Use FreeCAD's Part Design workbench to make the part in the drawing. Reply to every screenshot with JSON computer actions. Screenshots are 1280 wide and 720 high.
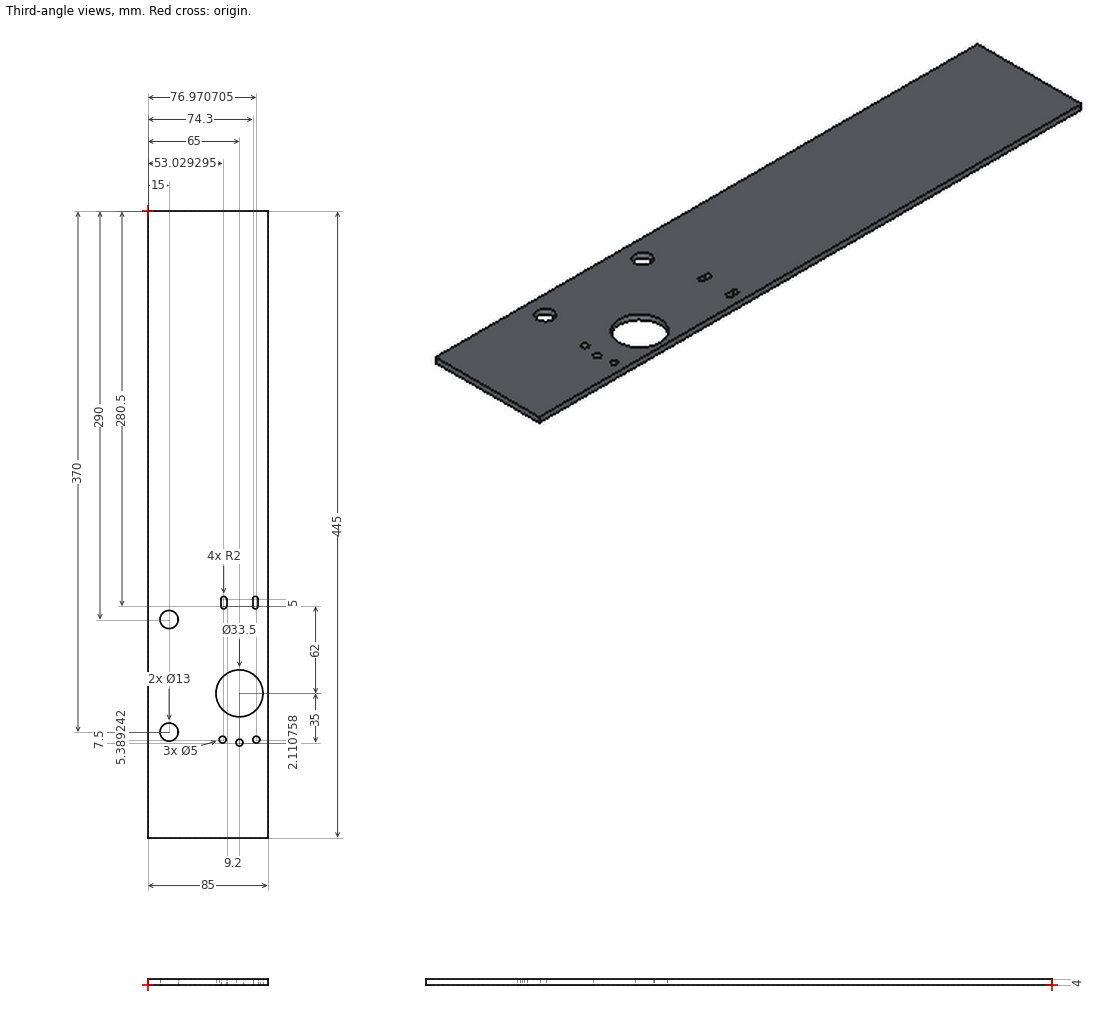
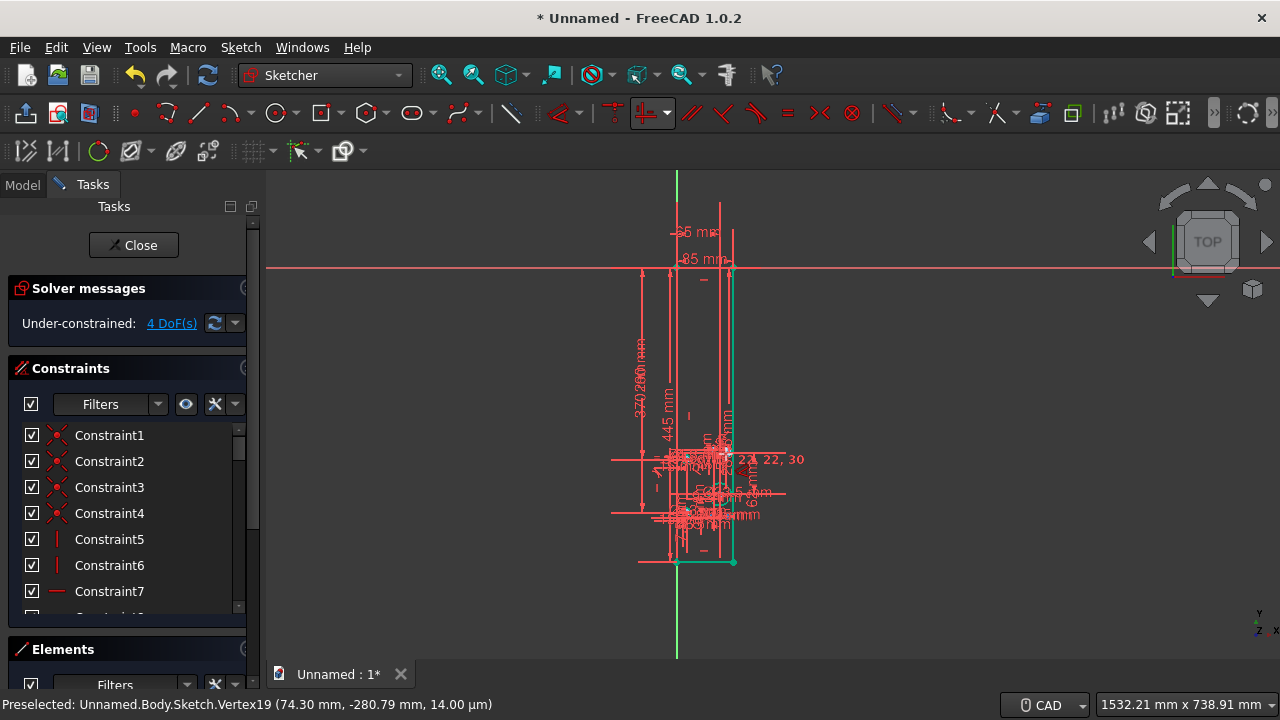
{"action": "scroll", "coordinate": [712, 517], "scroll_direction": "up", "scroll_amount": 3}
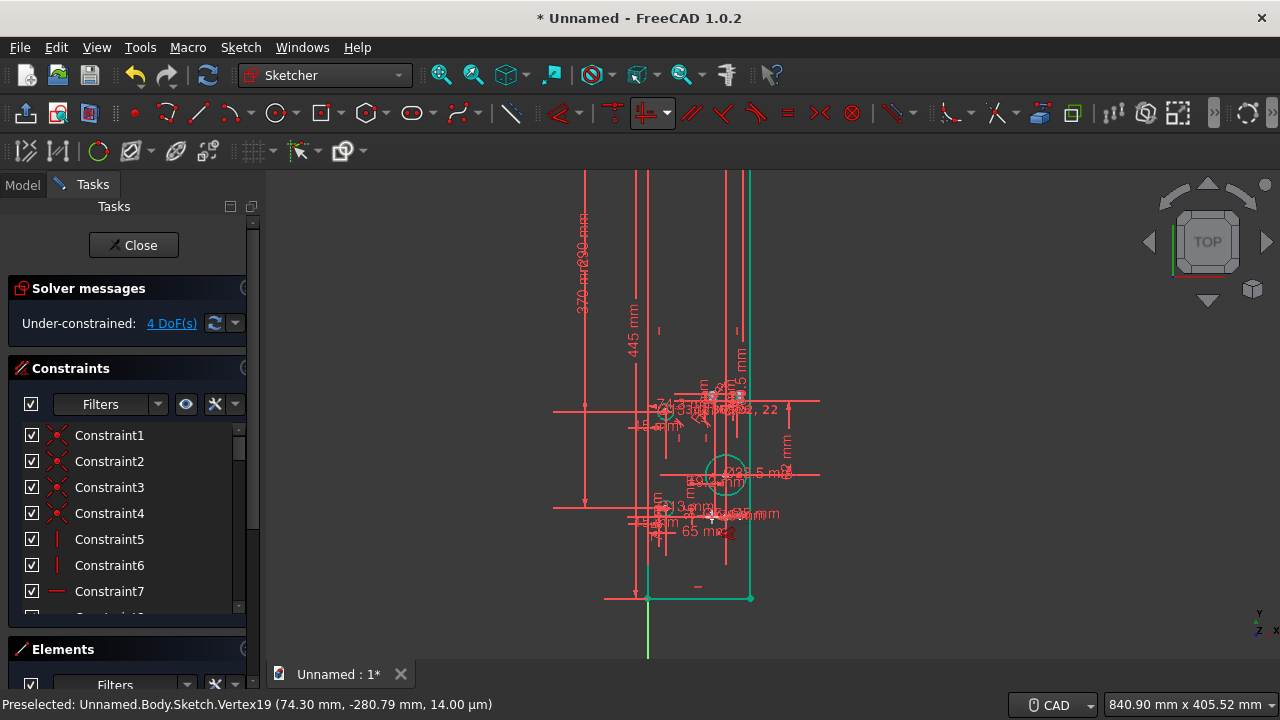
{"action": "left_click", "coordinate": [712, 516]}
{"action": "left_click", "coordinate": [680, 574]}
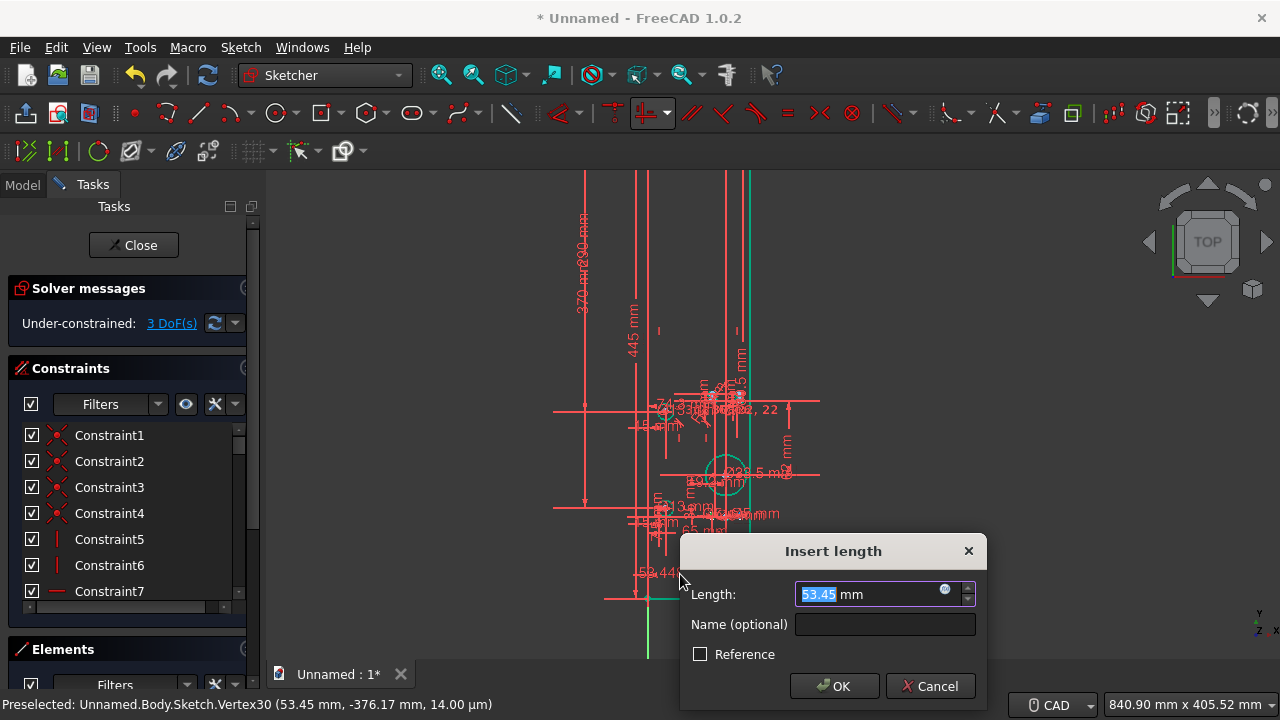
{"action": "type", "text": "53.029295"}
{"action": "key", "text": "Return"}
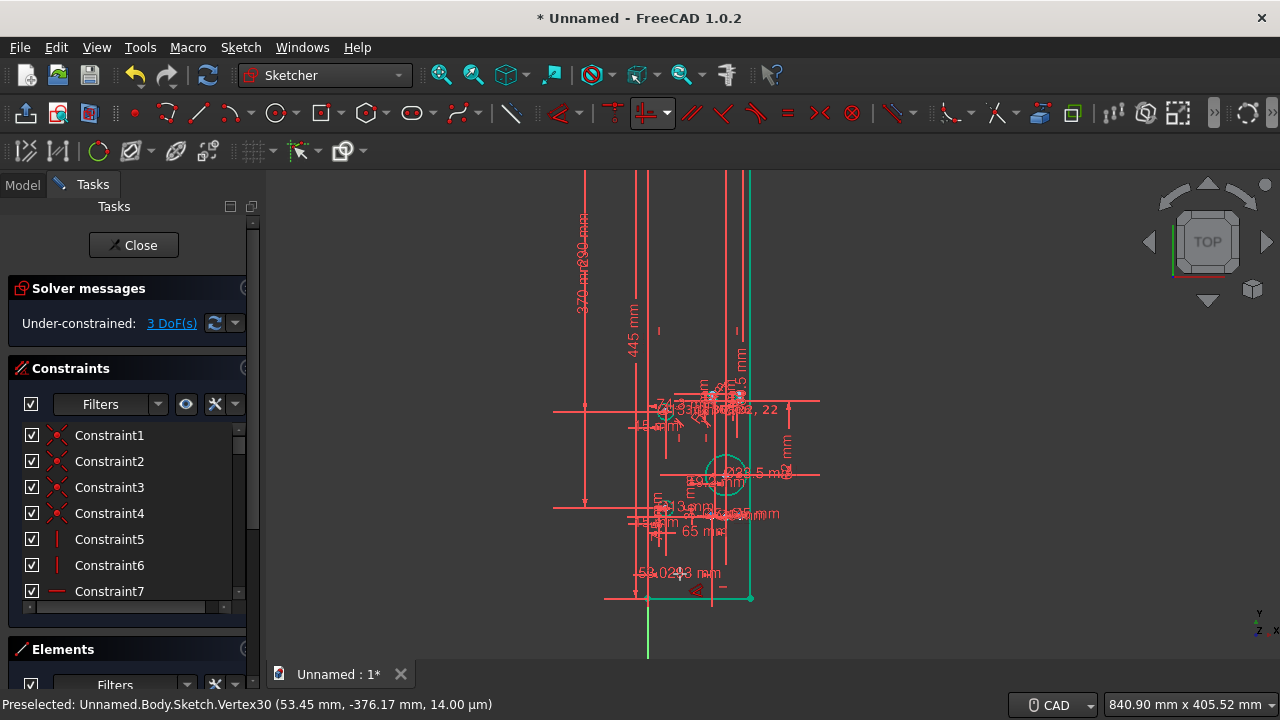
{"action": "left_click", "coordinate": [740, 516]}
{"action": "left_click", "coordinate": [694, 622]}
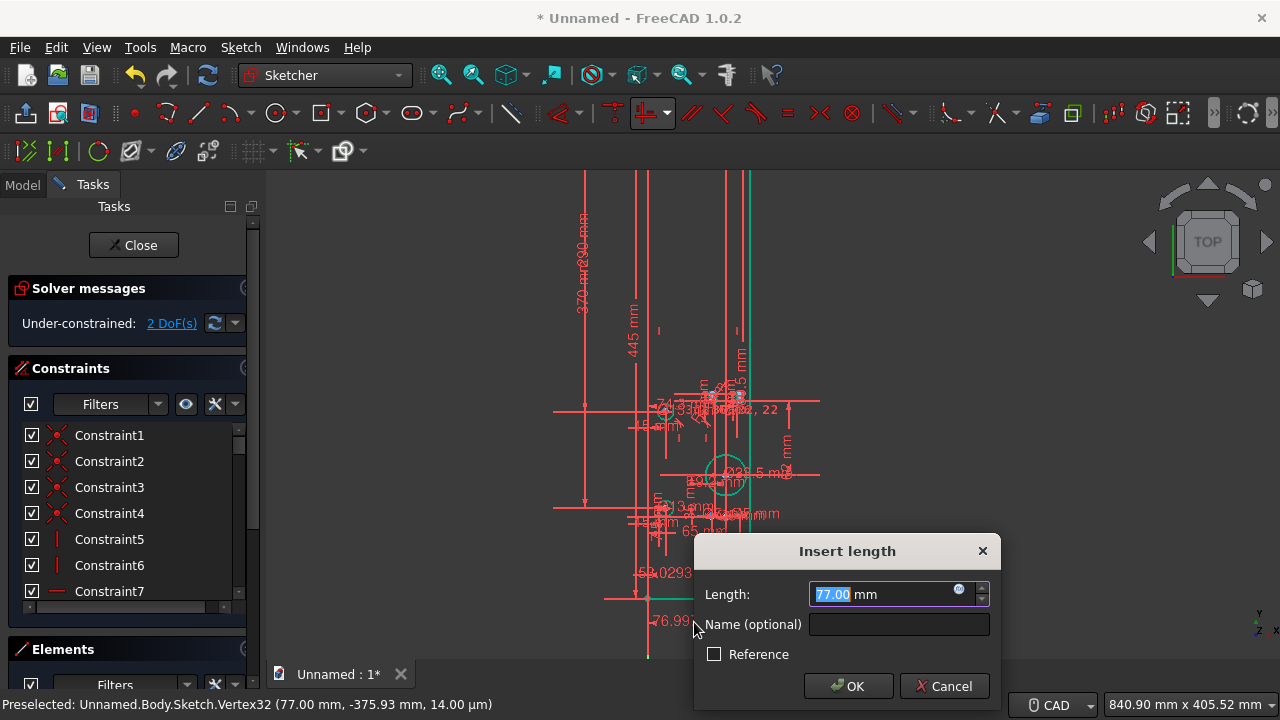
{"action": "type", "text": "76.970705"}
{"action": "key", "text": "Return"}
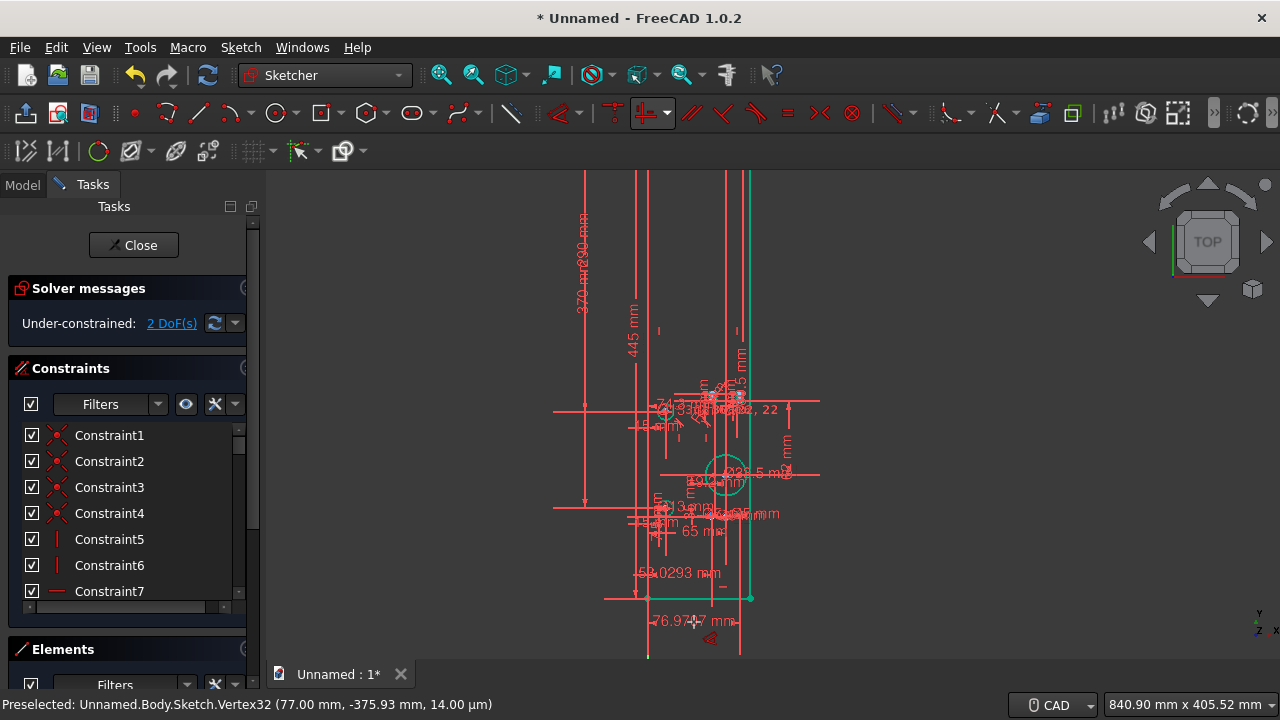
{"action": "scroll", "coordinate": [666, 508], "scroll_direction": "up", "scroll_amount": 10}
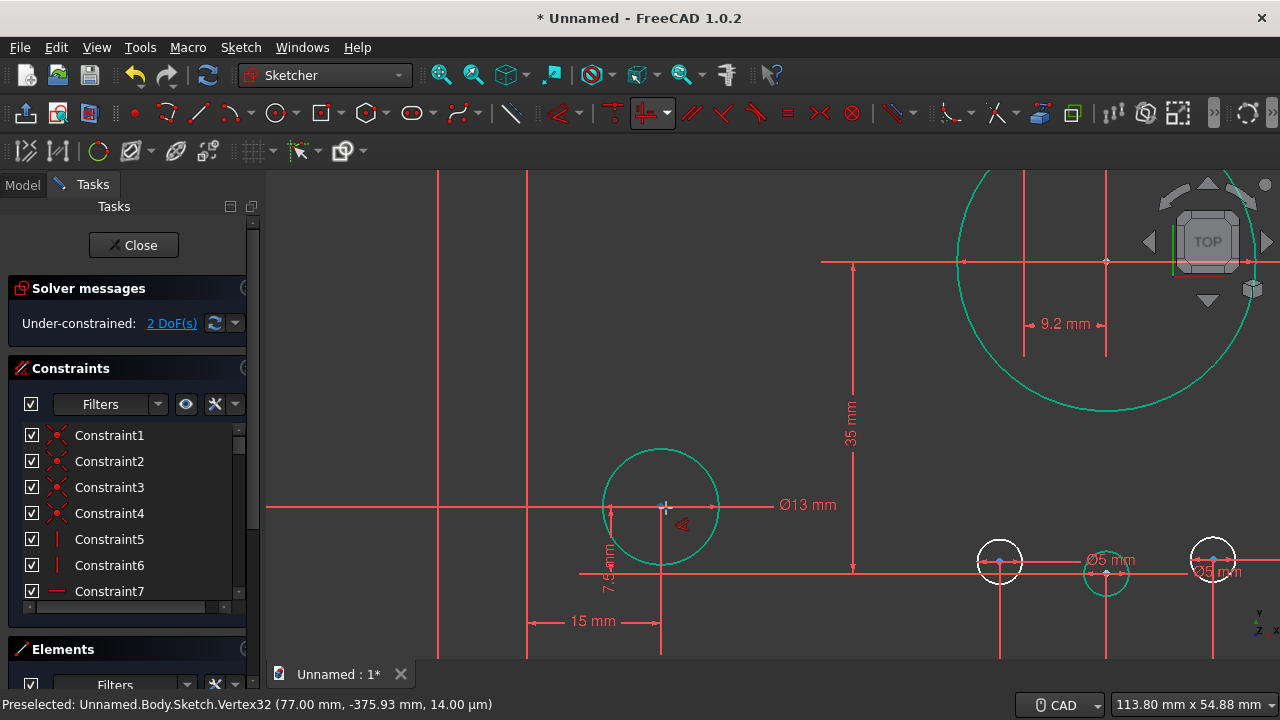
{"action": "left_click", "coordinate": [661, 507]}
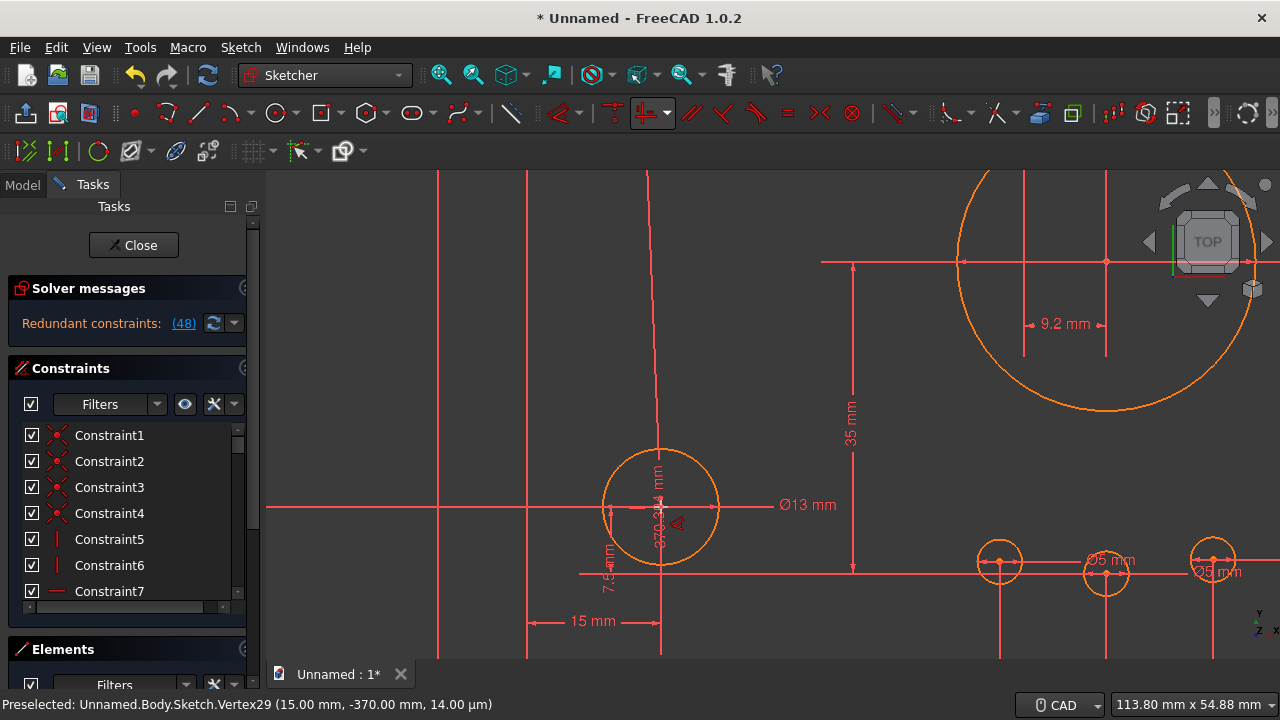
{"action": "left_click", "coordinate": [1000, 562]}
{"action": "left_click", "coordinate": [627, 534]}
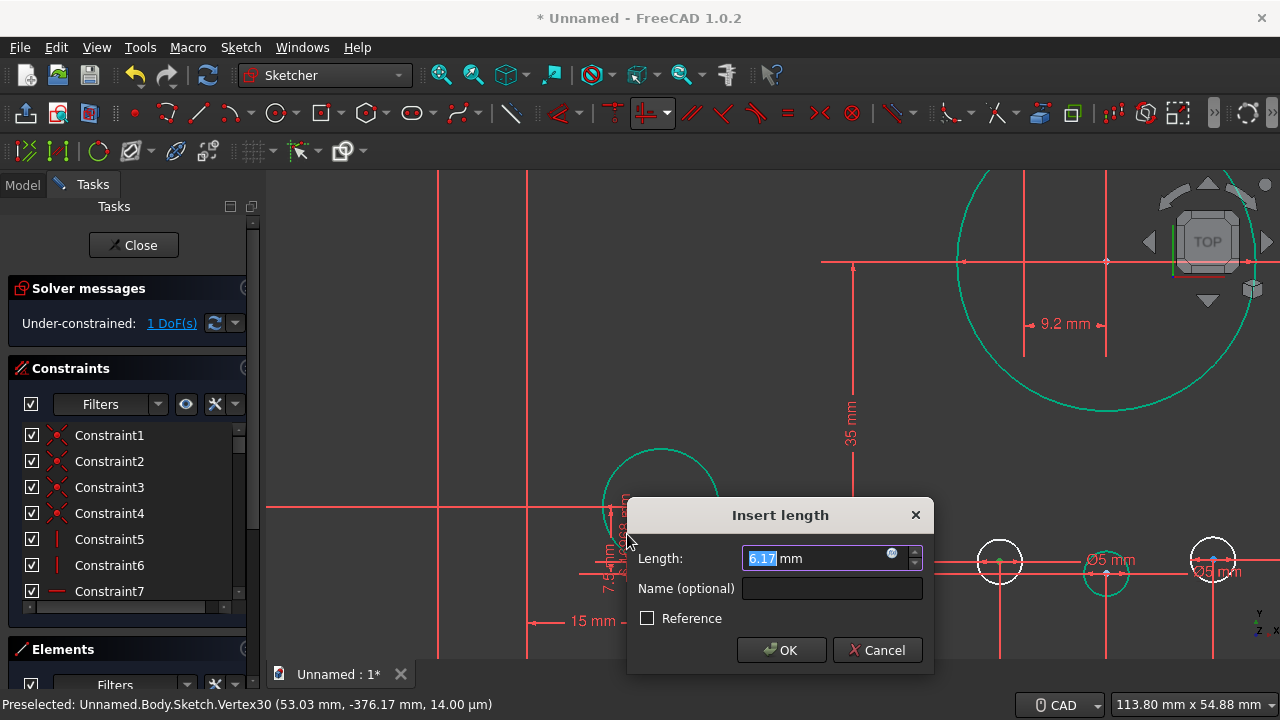
{"action": "type", "text": "5.389242"}
{"action": "key", "text": "Return"}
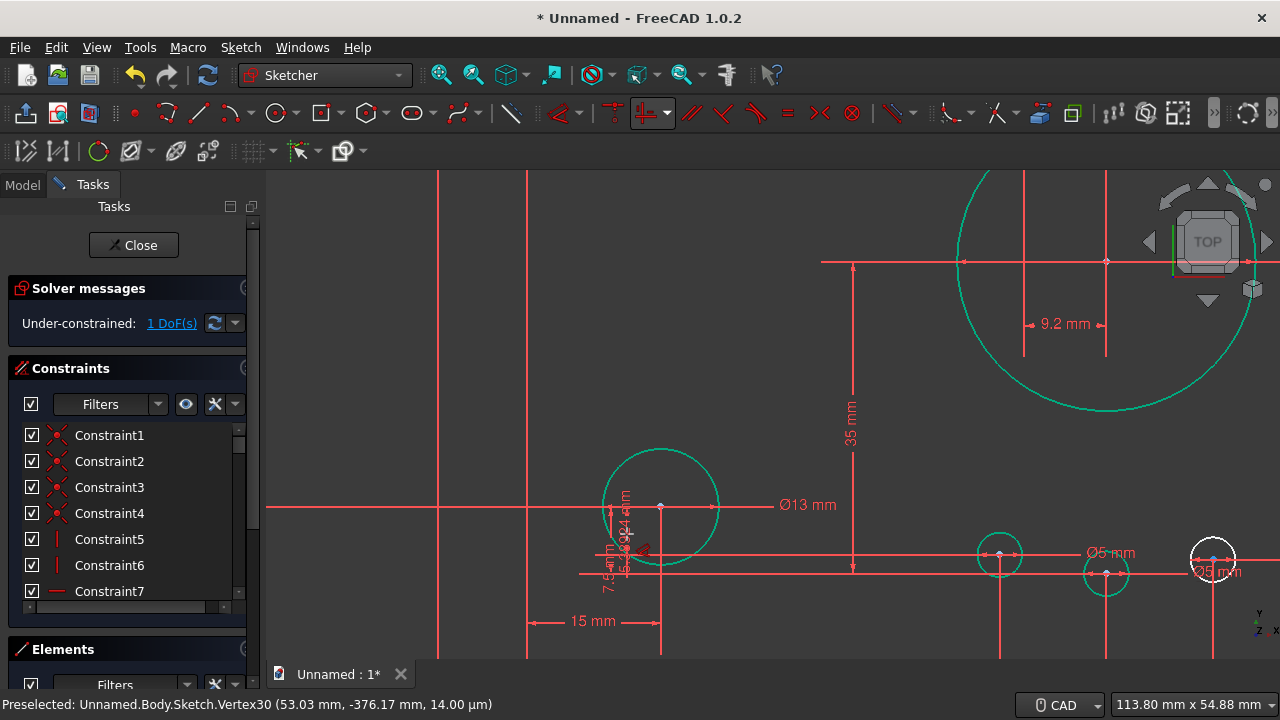
{"action": "scroll", "coordinate": [1106, 574], "scroll_direction": "up", "scroll_amount": 4}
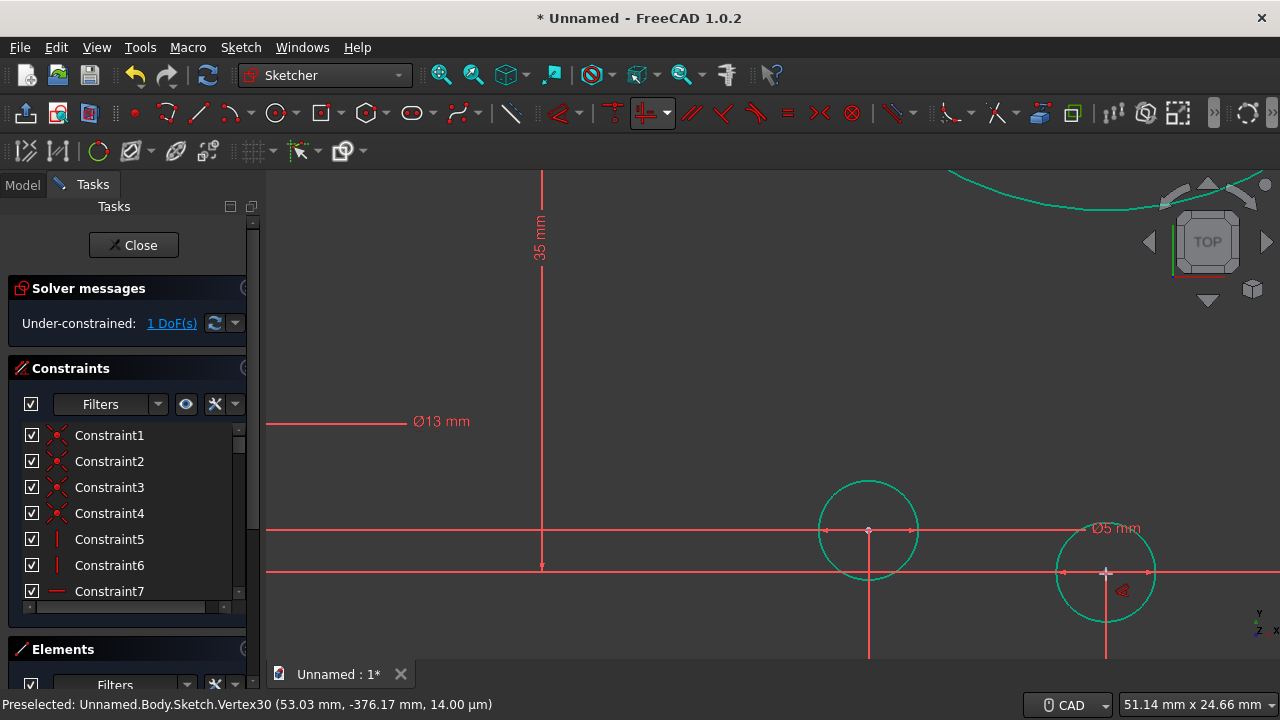
{"action": "left_click", "coordinate": [1106, 572]}